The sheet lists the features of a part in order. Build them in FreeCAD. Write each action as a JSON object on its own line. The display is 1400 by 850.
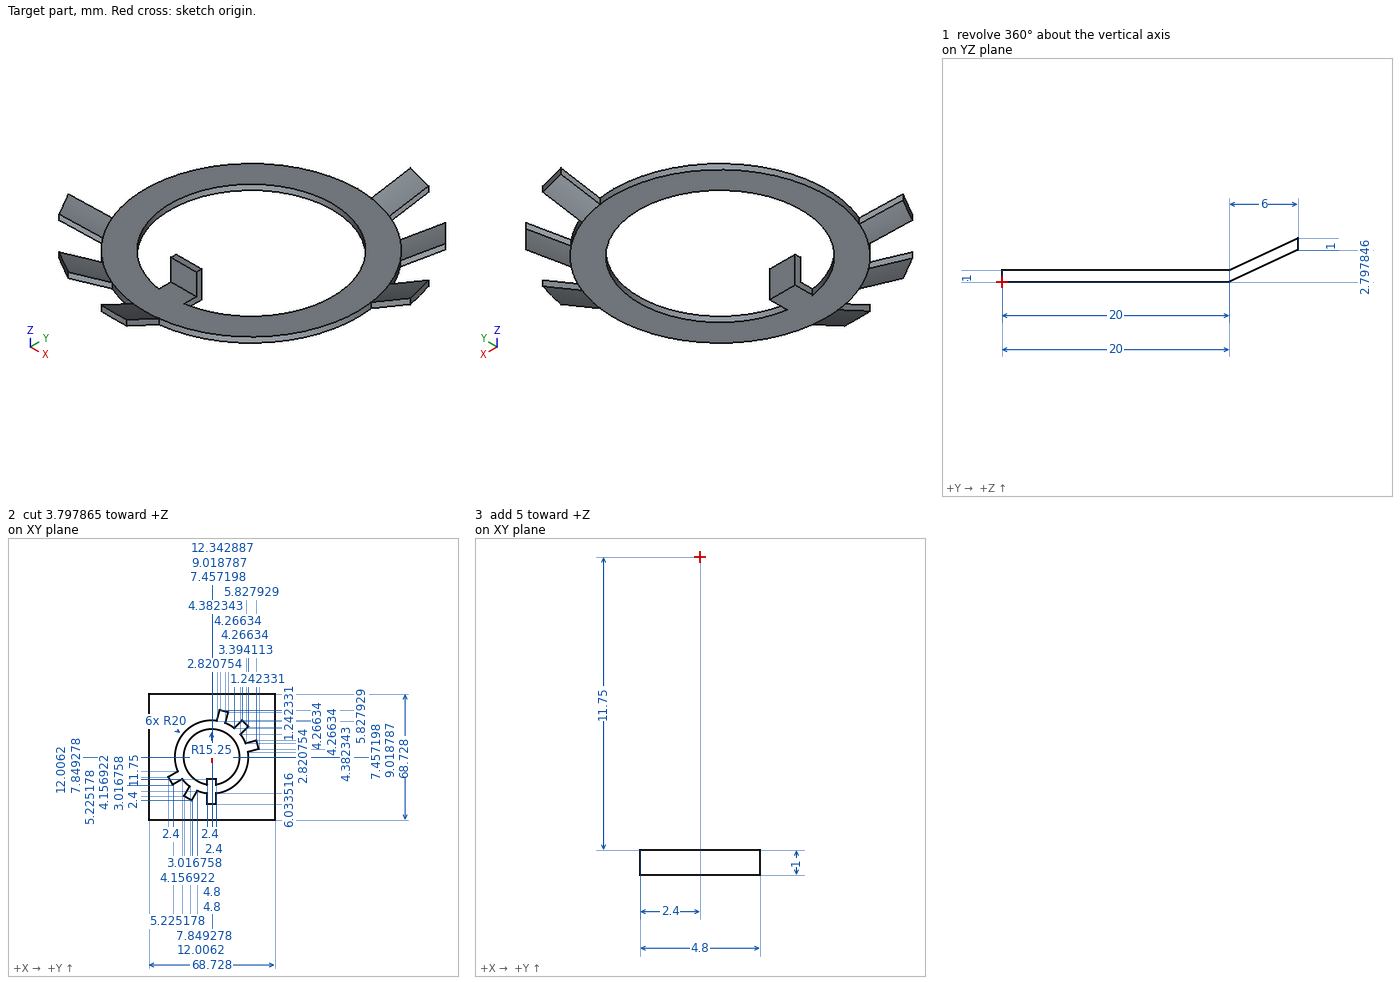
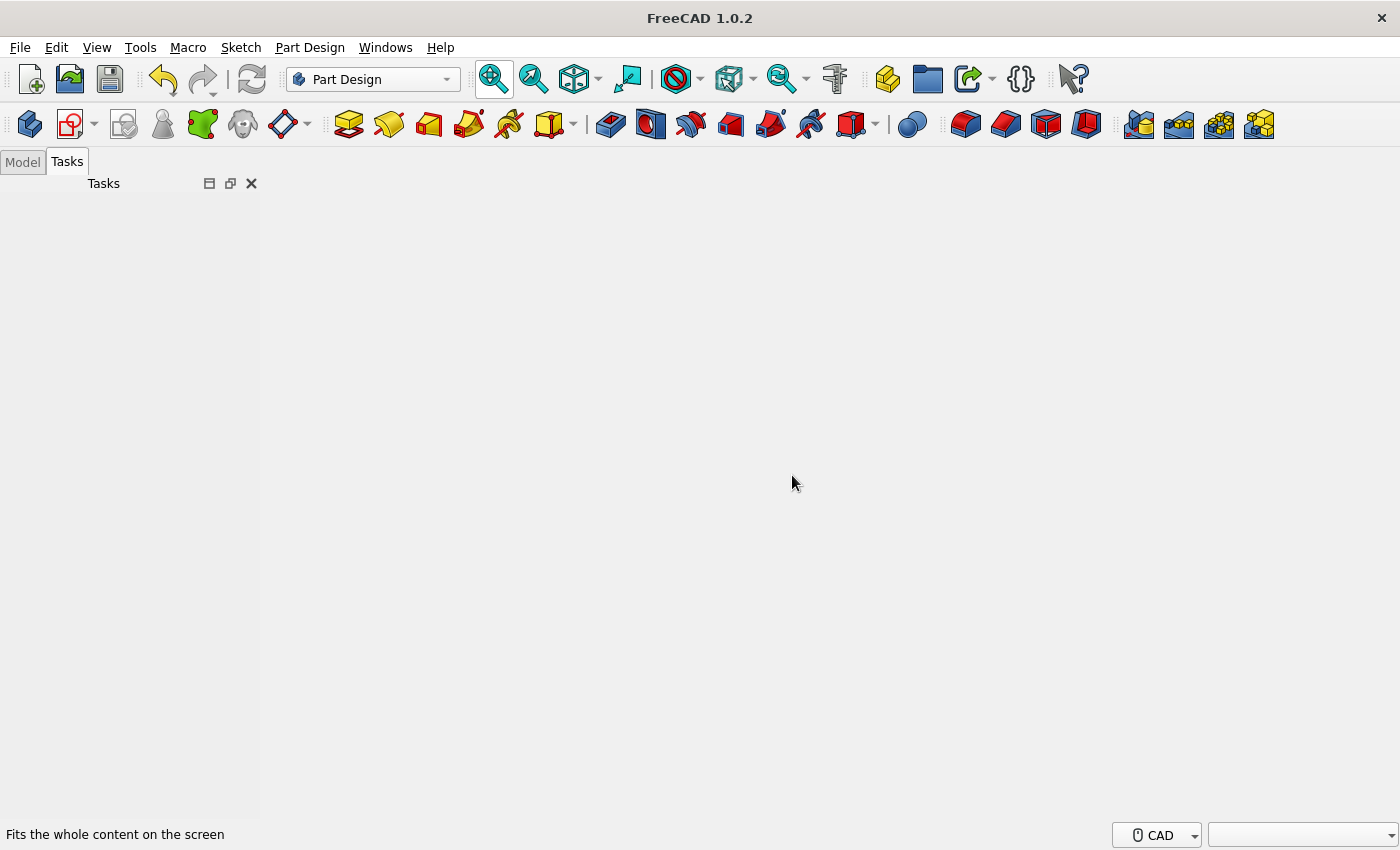
{"action": "left_click", "coordinate": [30, 80]}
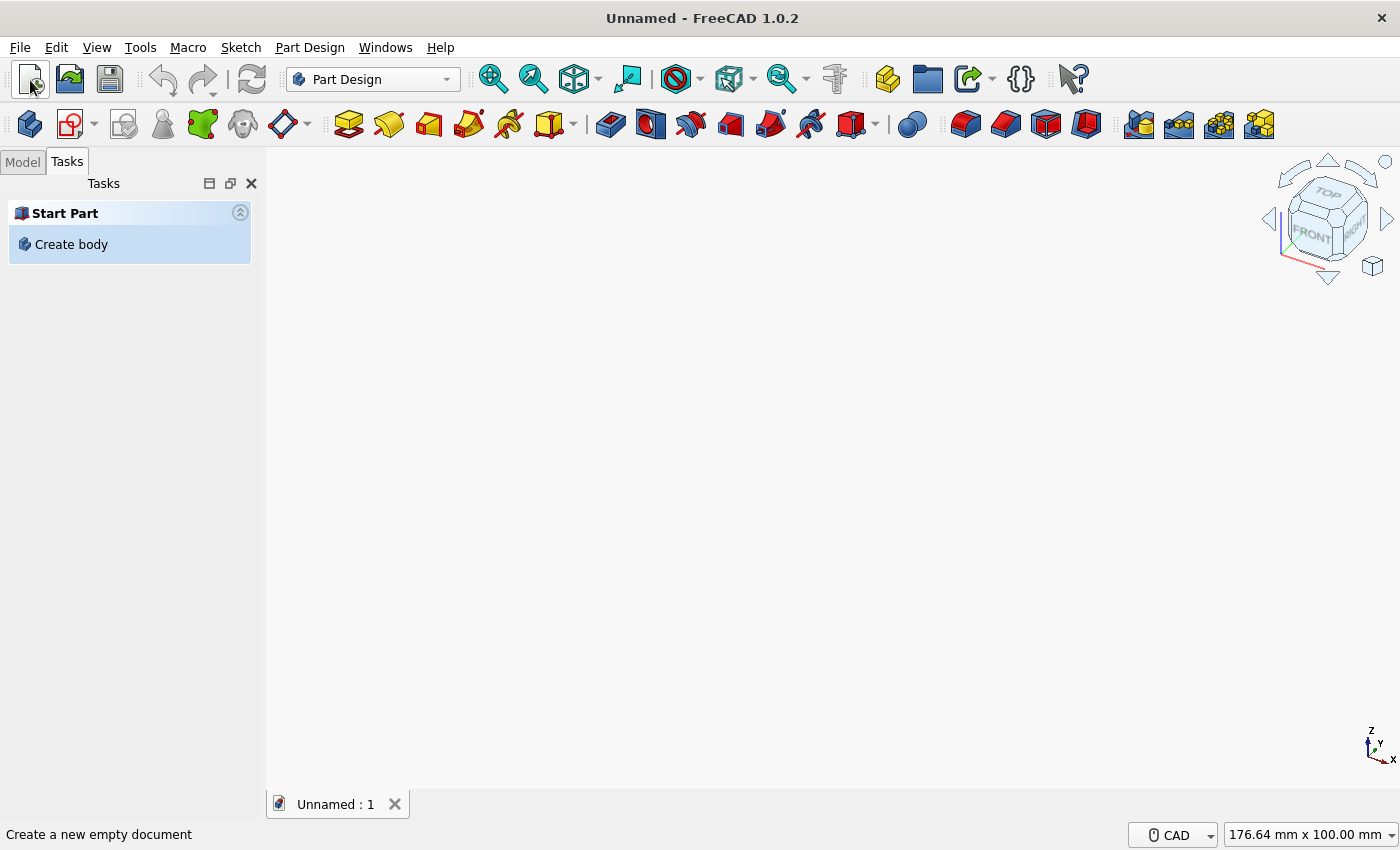
{"action": "left_click", "coordinate": [70, 124]}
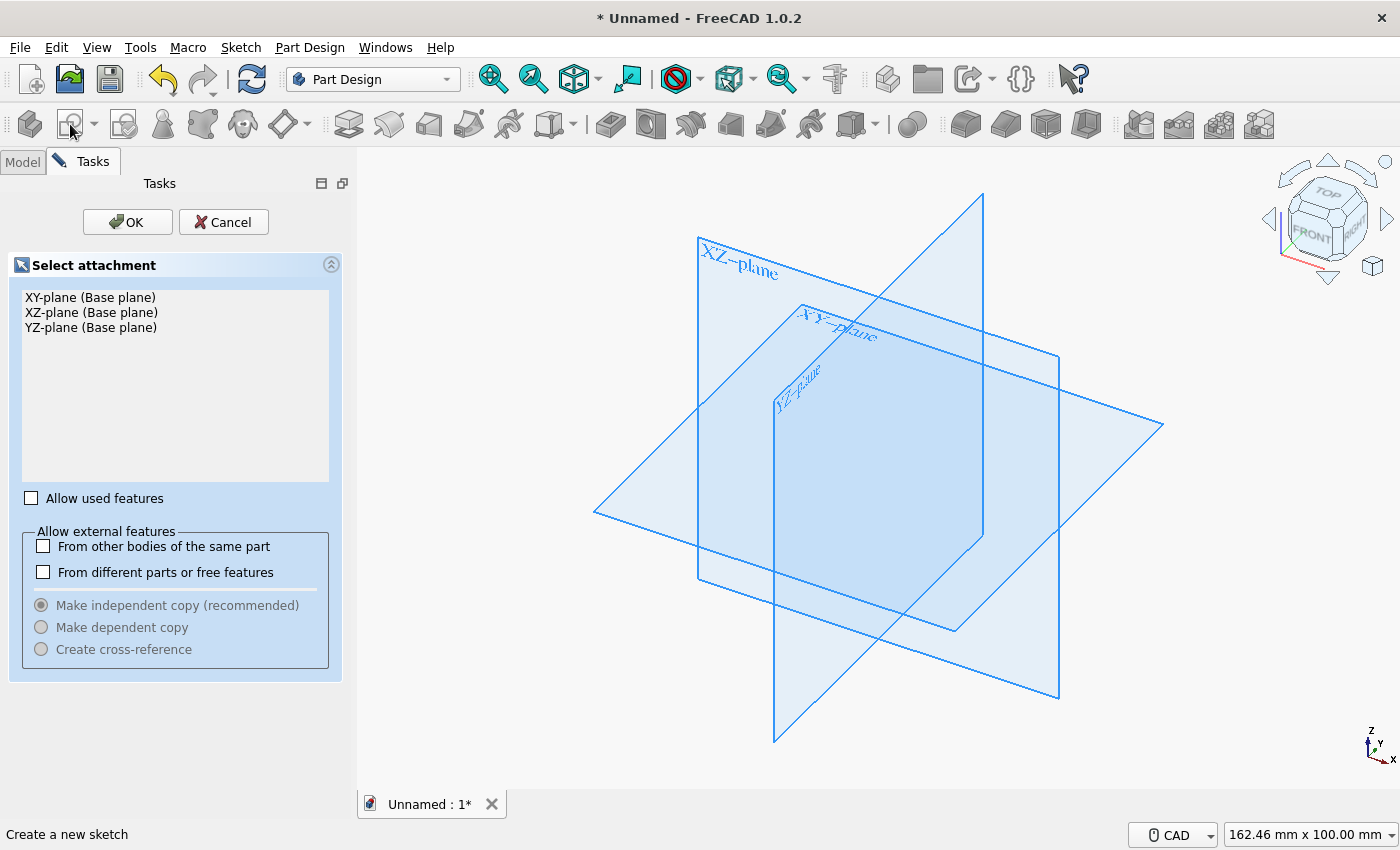
{"action": "left_click", "coordinate": [82, 328]}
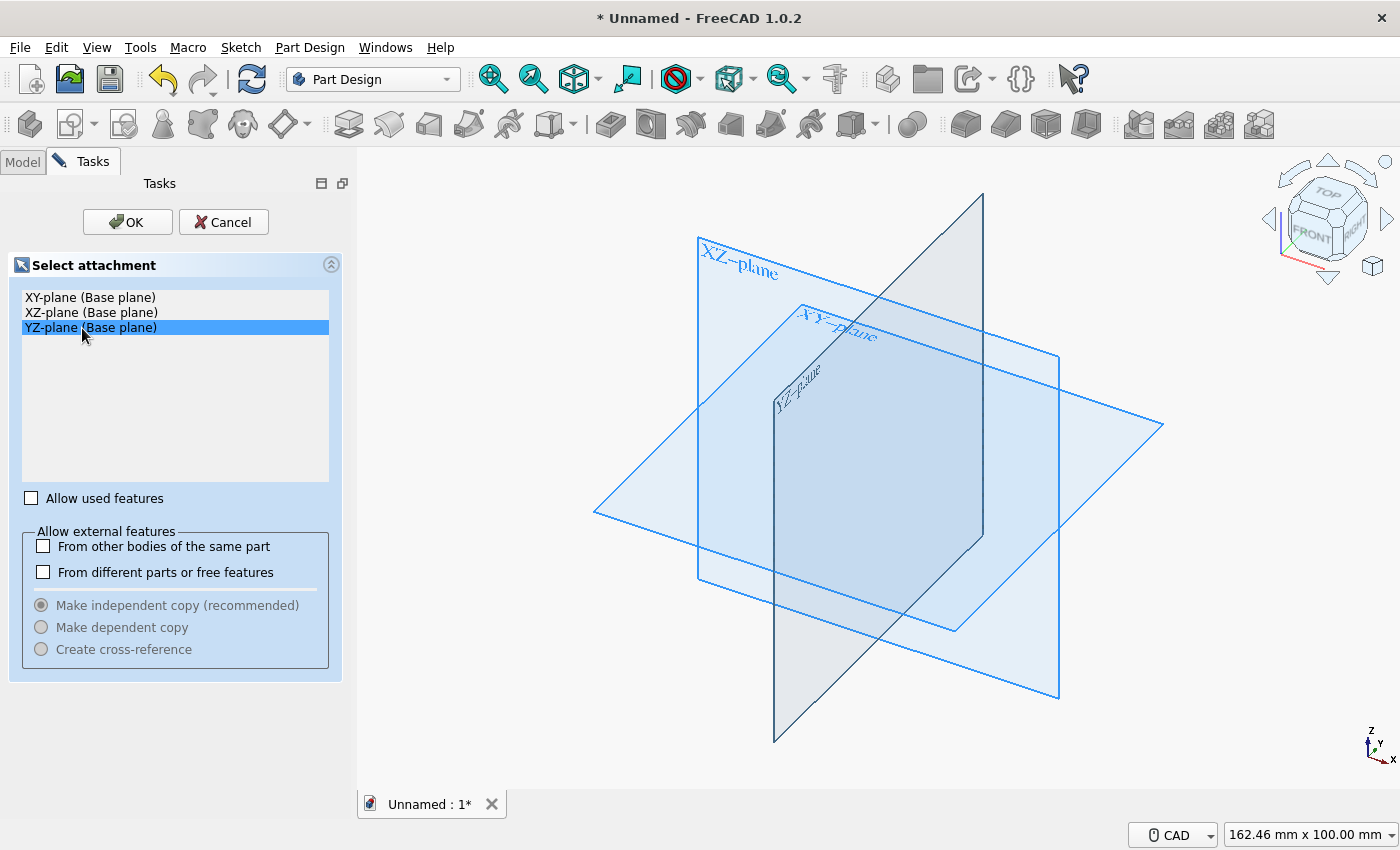
{"action": "left_click", "coordinate": [128, 222]}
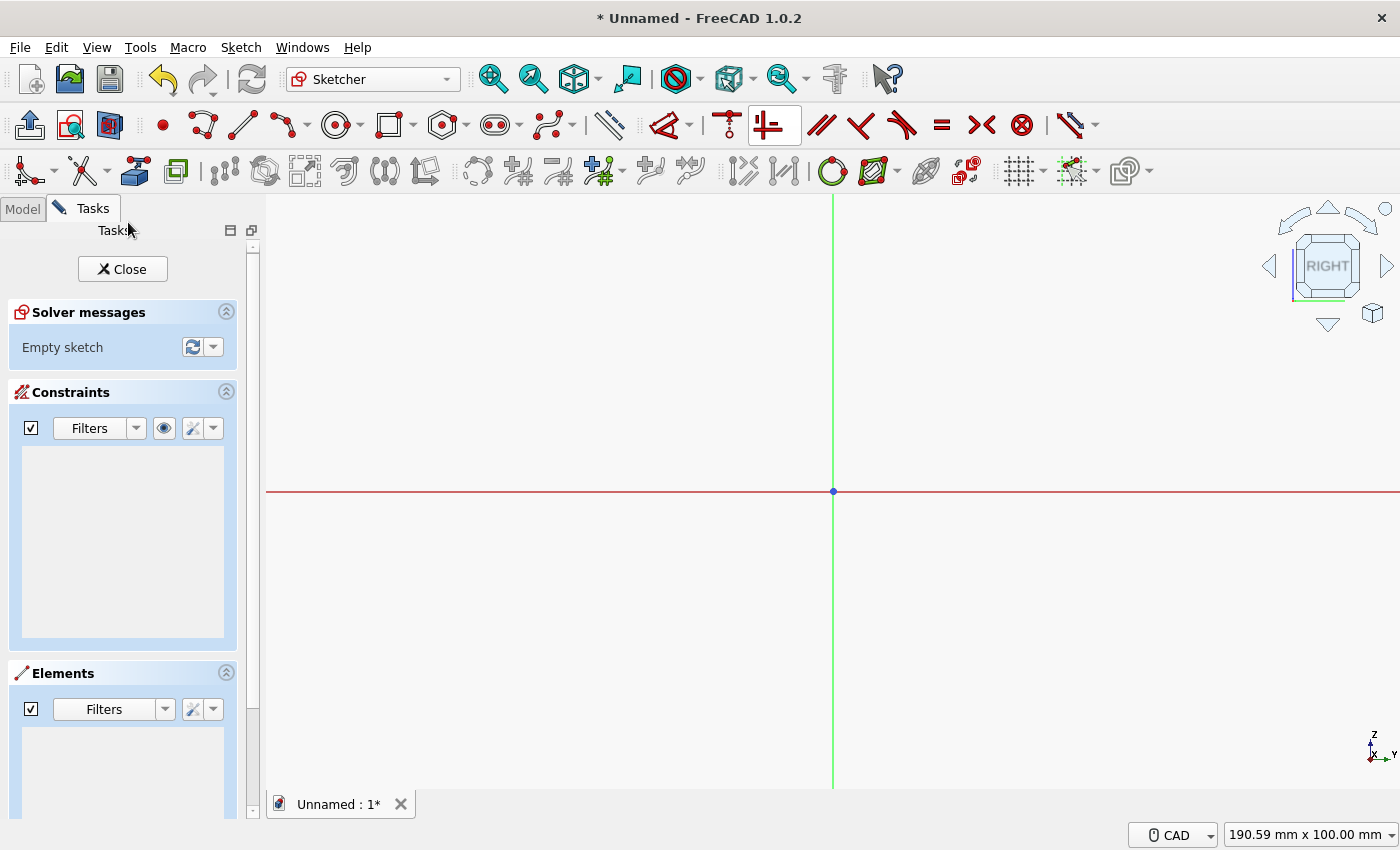
{"action": "scroll", "coordinate": [958, 477], "scroll_direction": "up", "scroll_amount": 7}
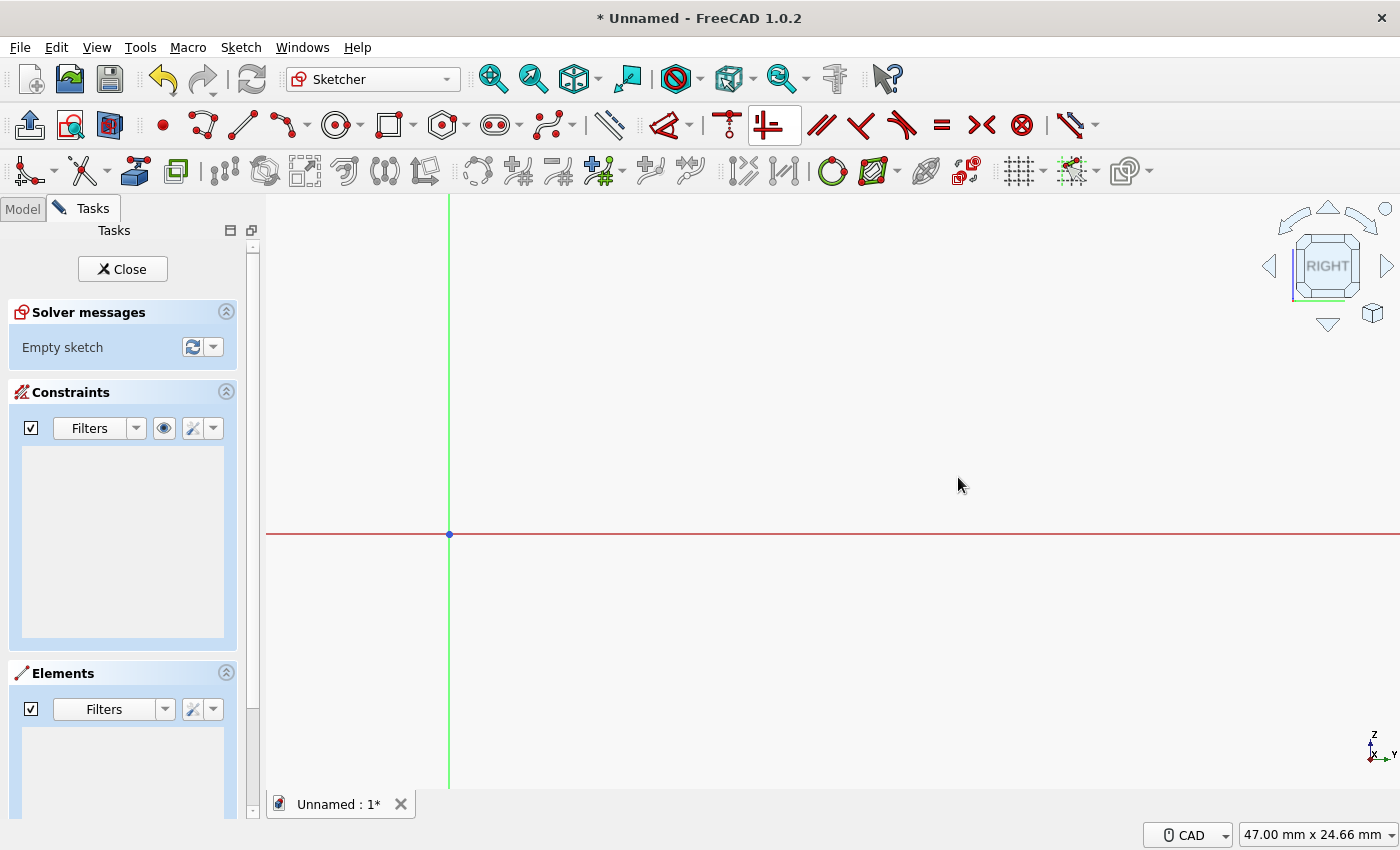
{"action": "left_click", "coordinate": [204, 126]}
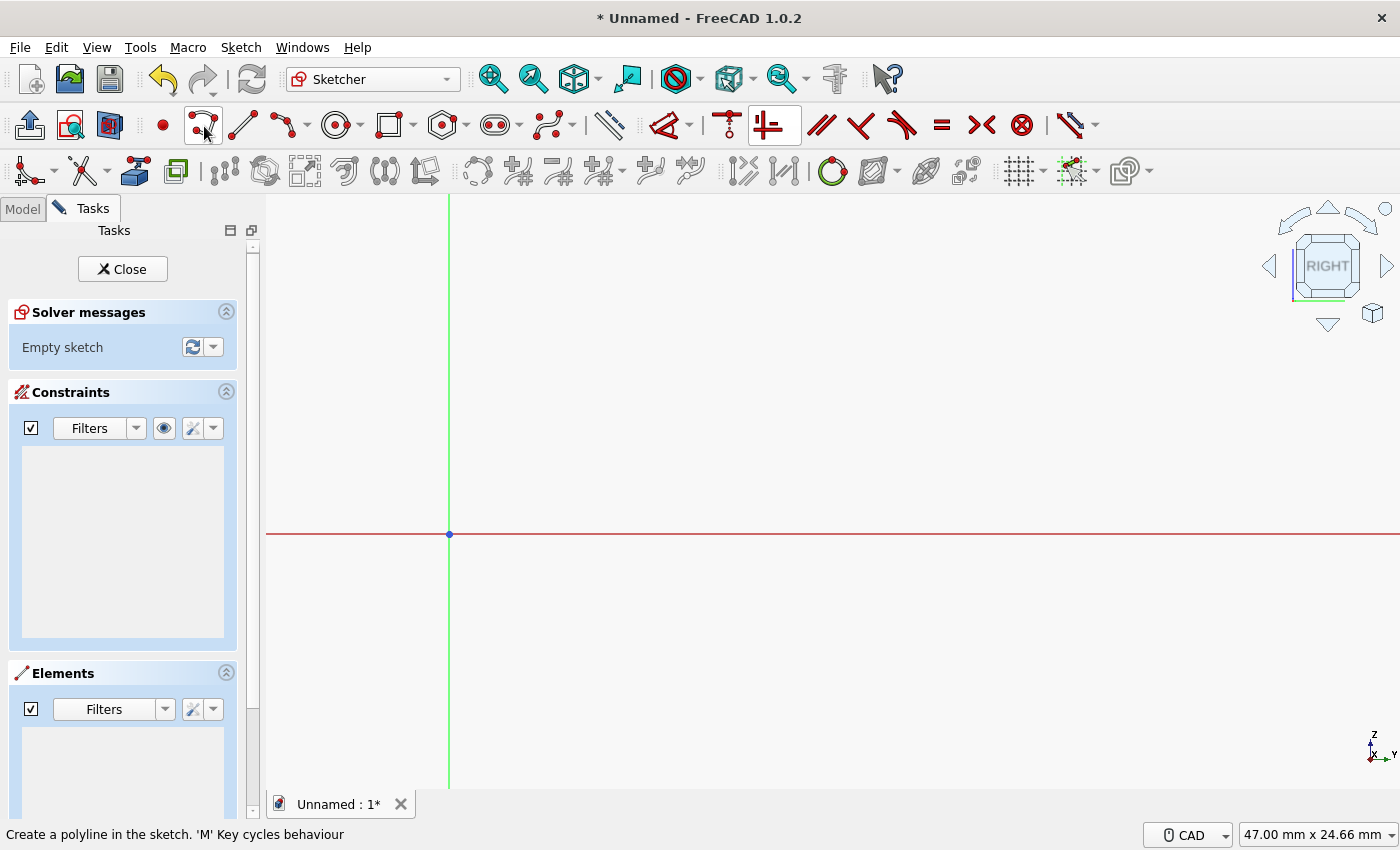
{"action": "left_click", "coordinate": [449, 534]}
{"action": "left_click", "coordinate": [932, 525]}
{"action": "left_click", "coordinate": [1077, 467]}
{"action": "left_click", "coordinate": [1077, 443]}
{"action": "left_click", "coordinate": [932, 510]}
{"action": "left_click", "coordinate": [458, 510]}
{"action": "left_click", "coordinate": [449, 534]}
{"action": "key", "text": "Escape"}
{"action": "key", "text": "Escape"}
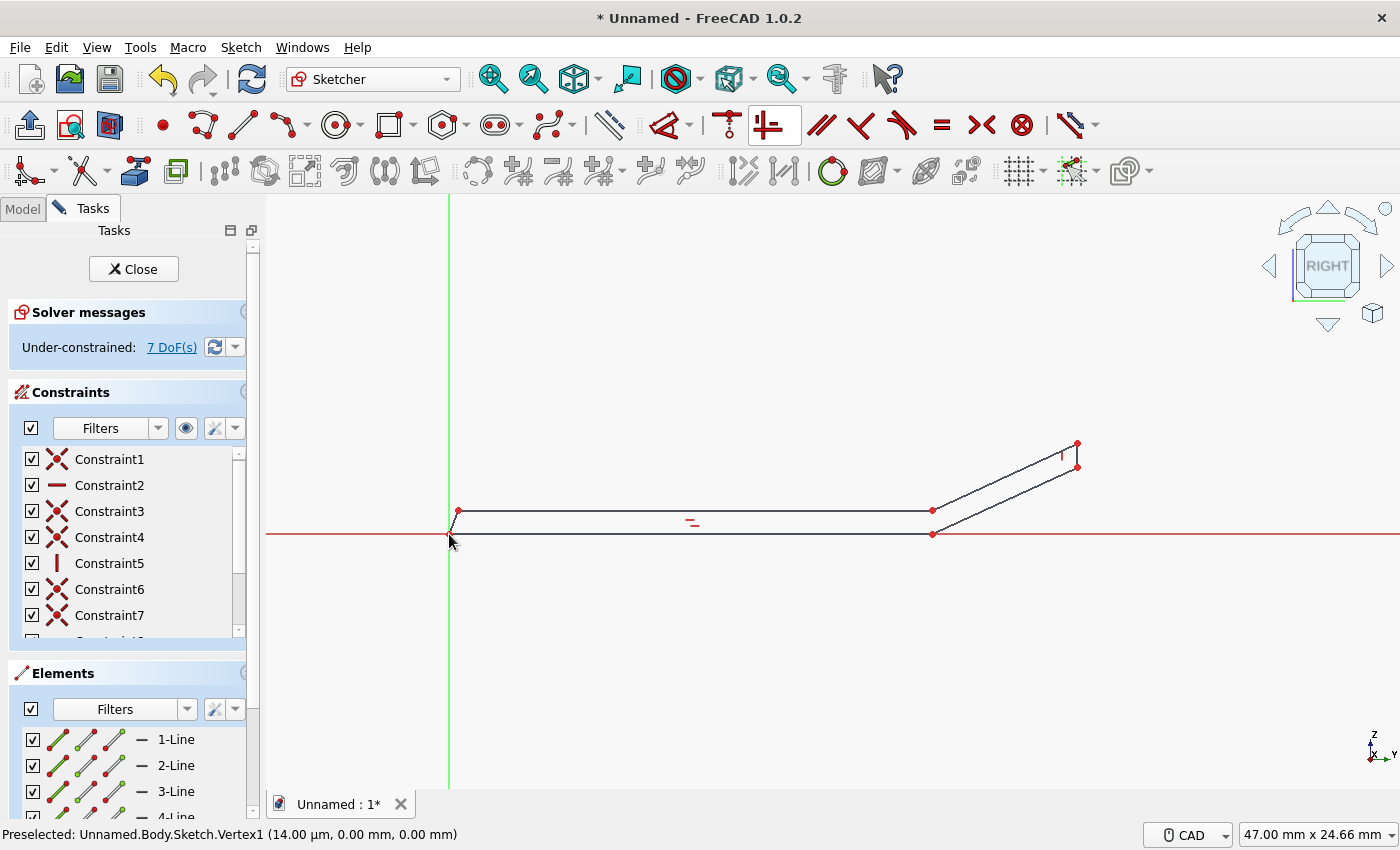
{"action": "scroll", "coordinate": [453, 525], "scroll_direction": "up", "scroll_amount": 2}